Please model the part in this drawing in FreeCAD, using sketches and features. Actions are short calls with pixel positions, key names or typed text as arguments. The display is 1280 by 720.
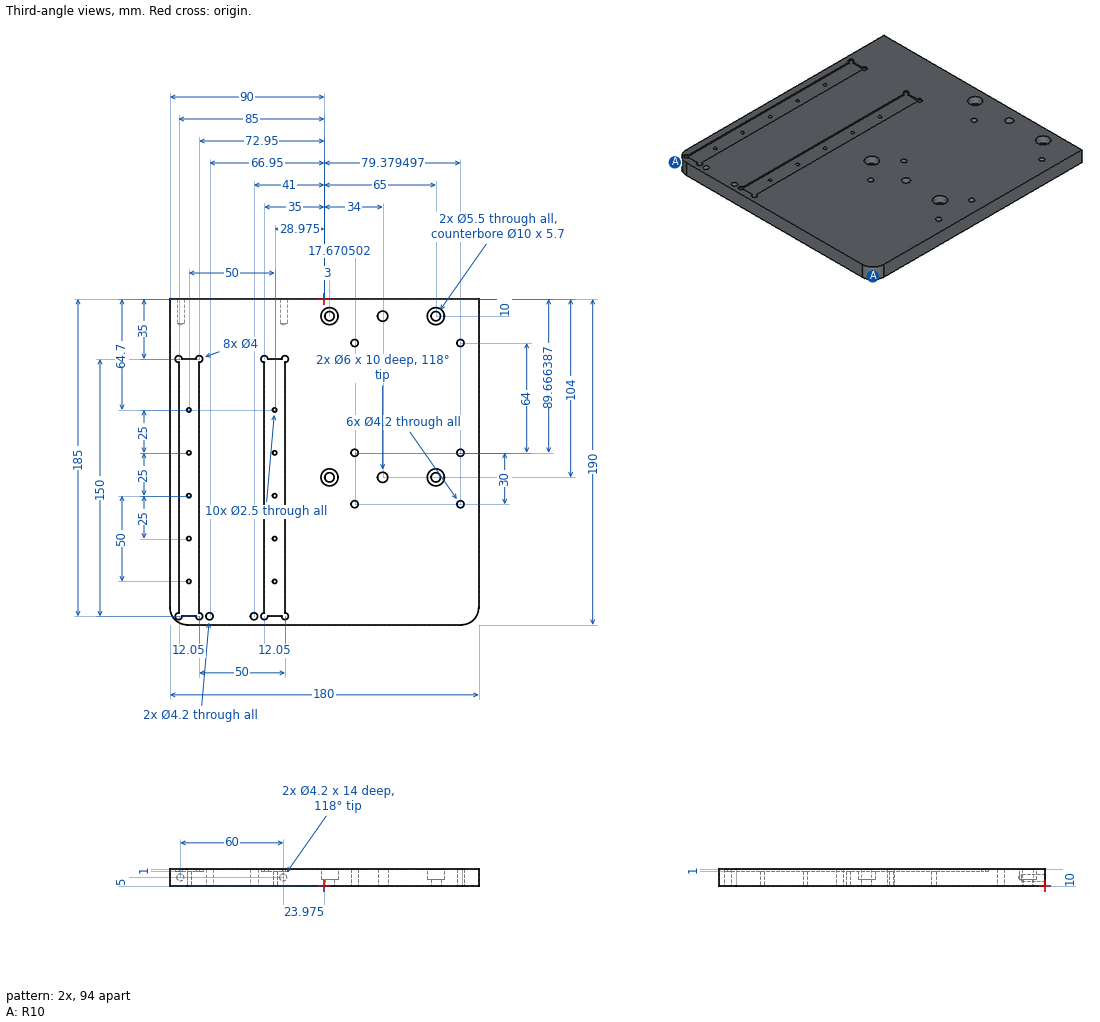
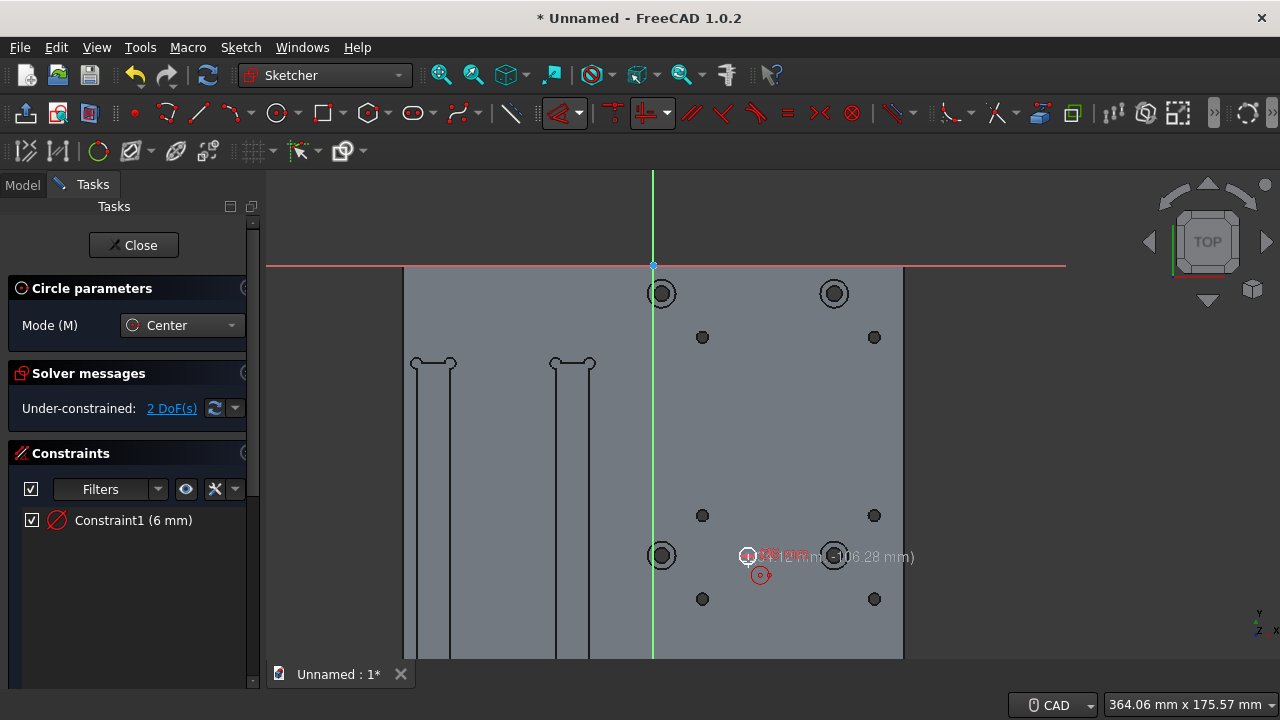
scroll(748, 294, up, 5)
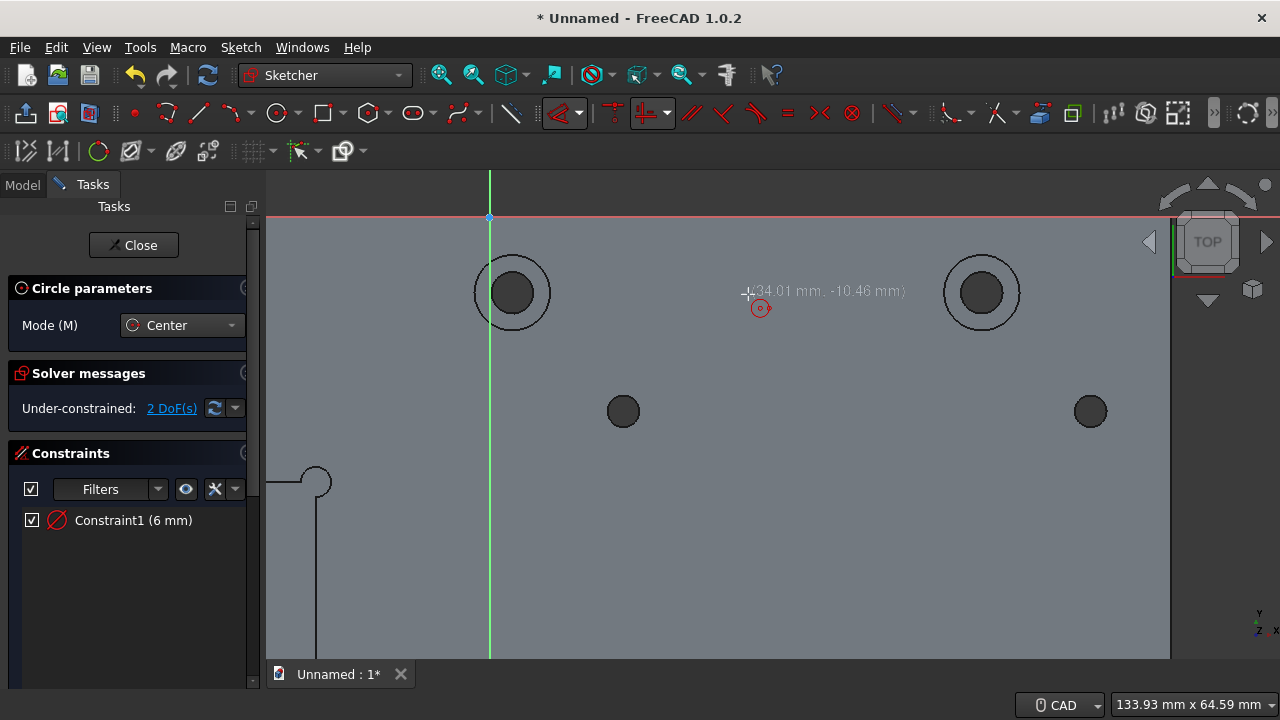
click(747, 293)
move(763, 277)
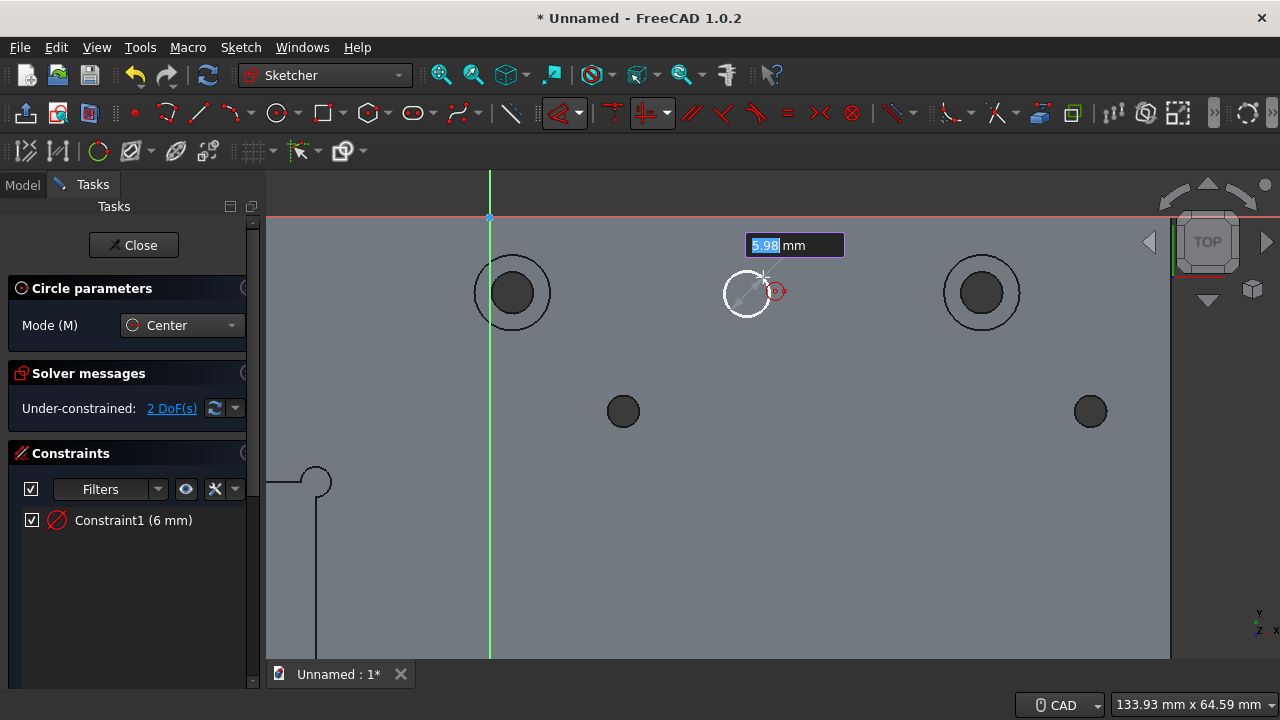
text(6)
key(Return)
key(Escape)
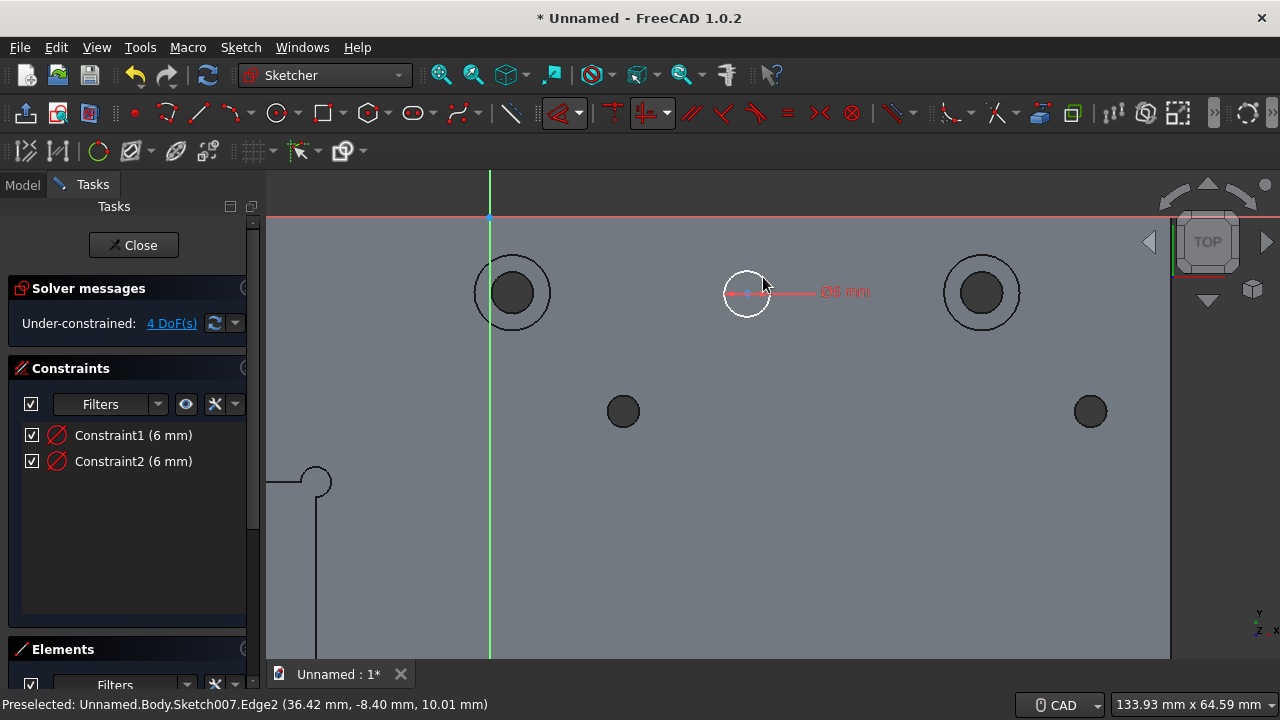
scroll(748, 294, down, 5)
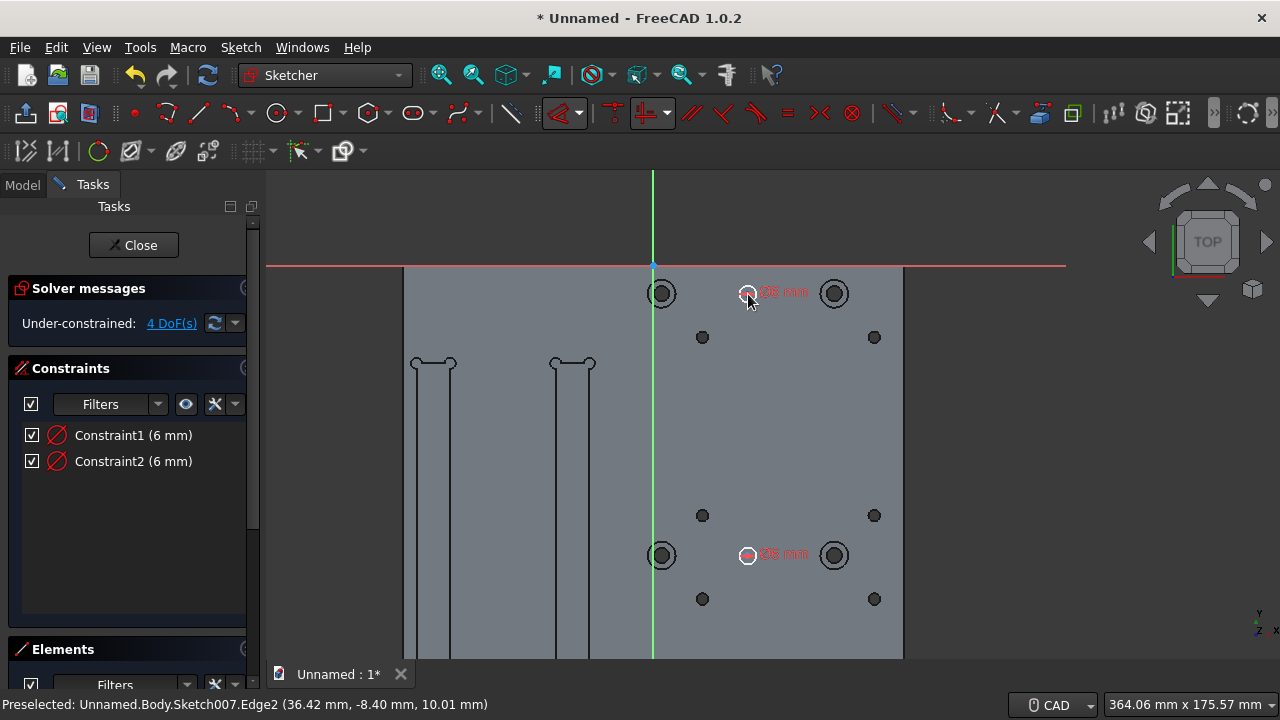
click(748, 556)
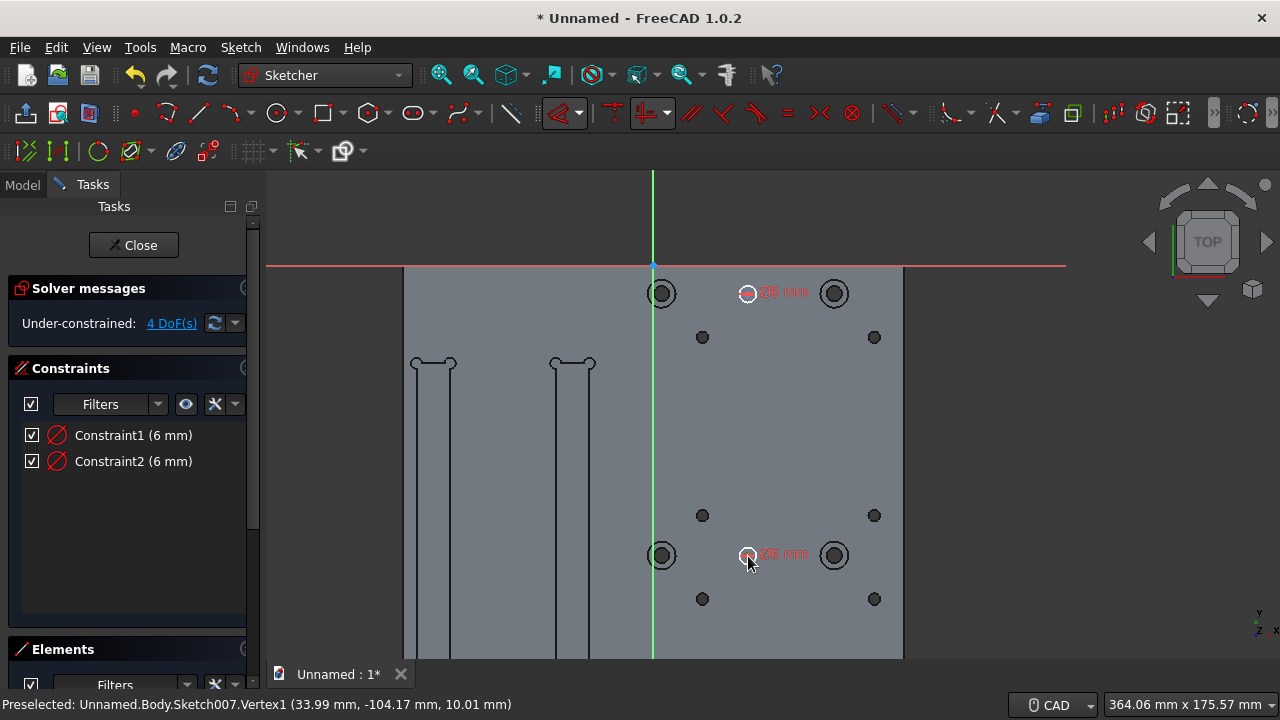
click(748, 294)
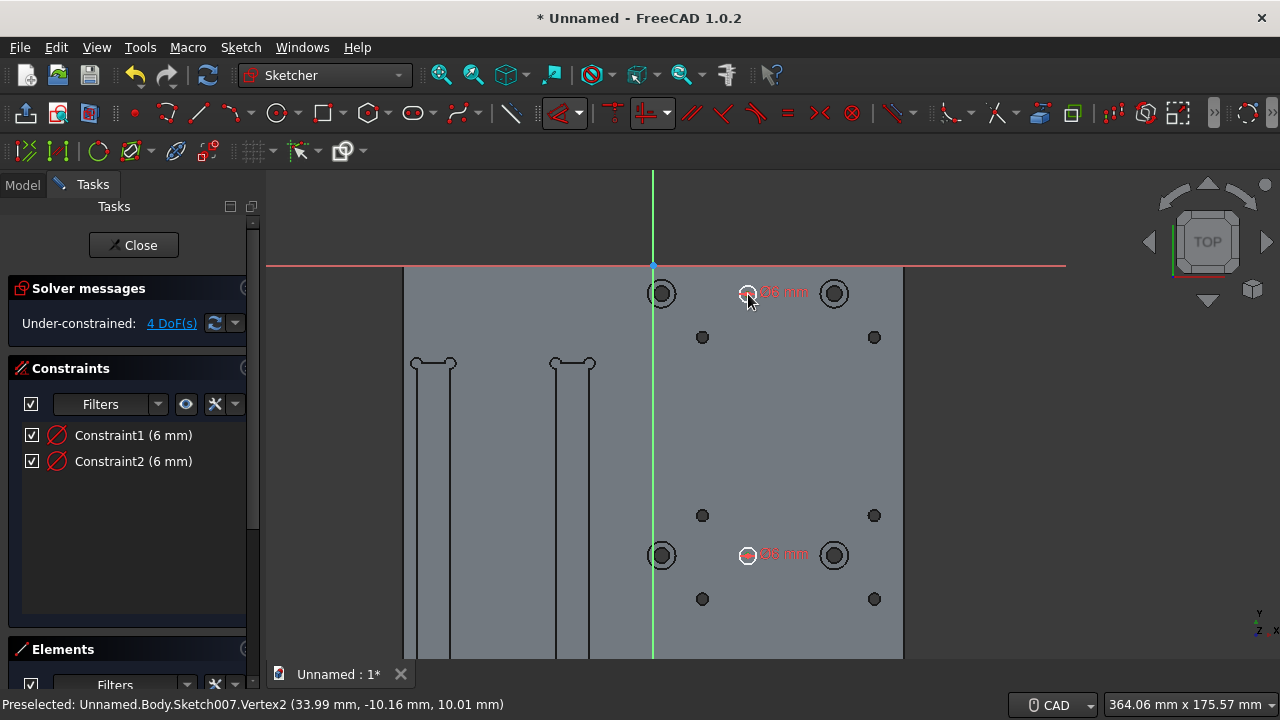
key(v)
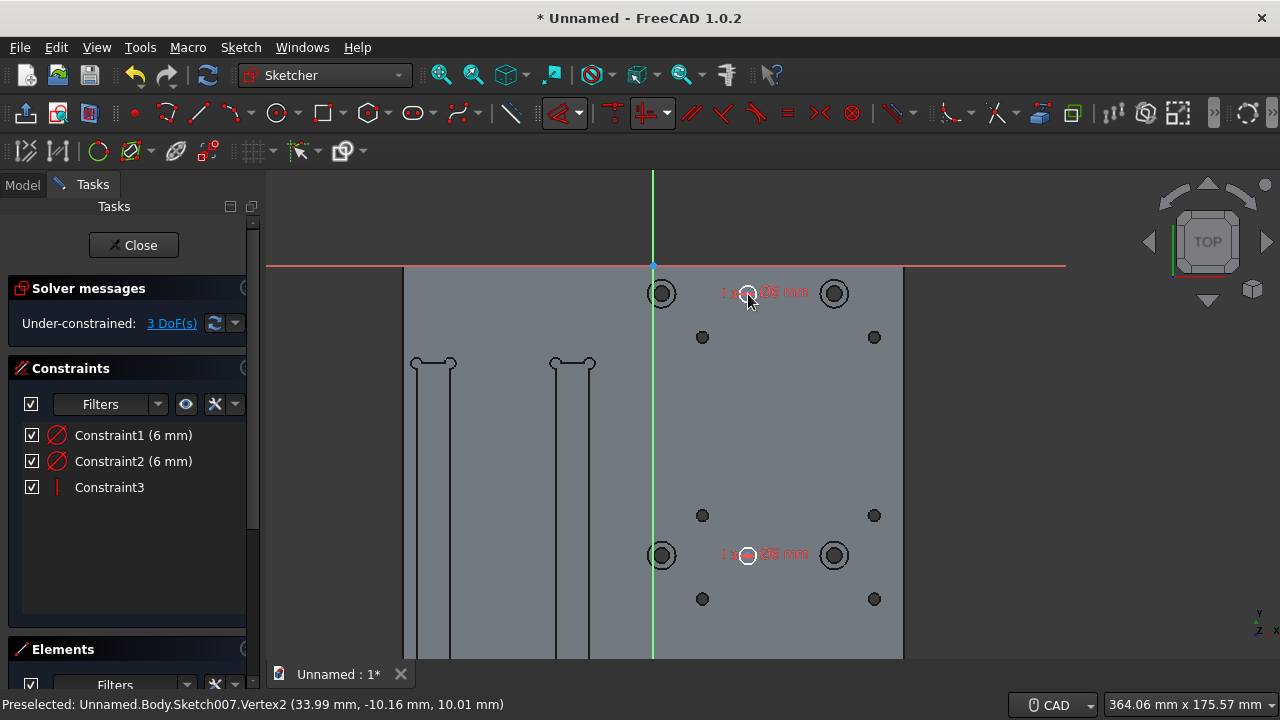
click(748, 556)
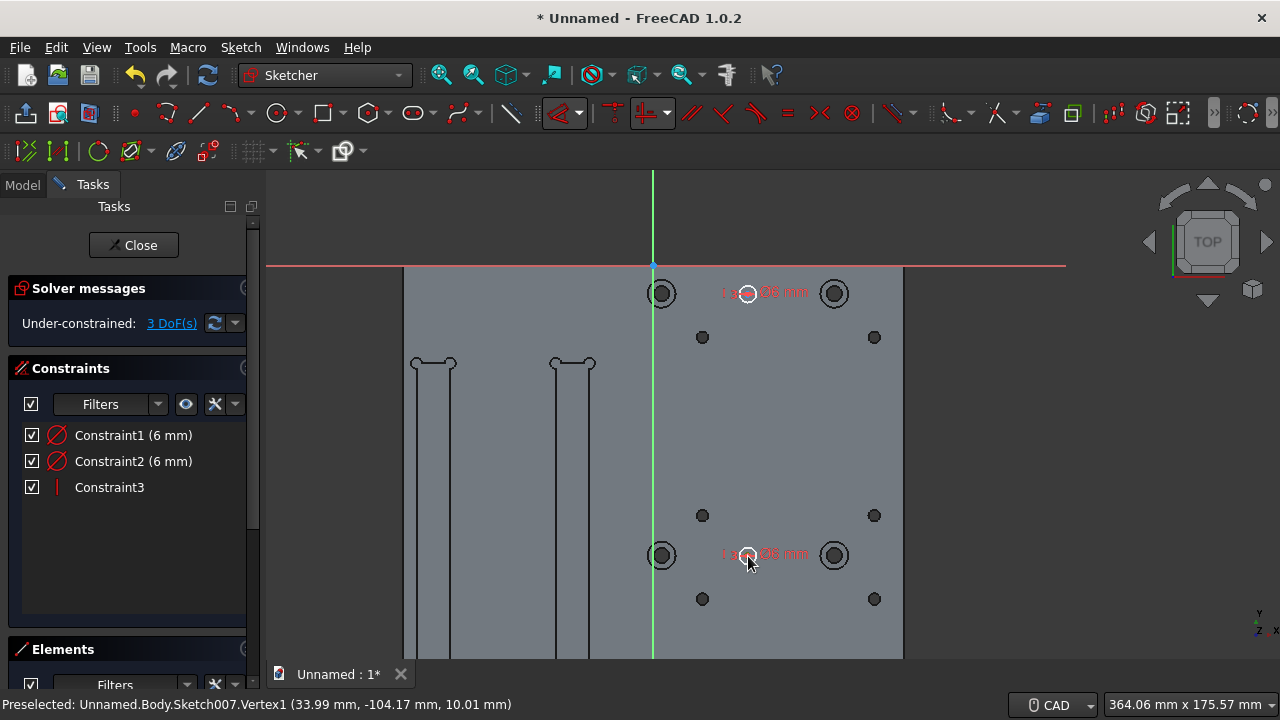
key(l)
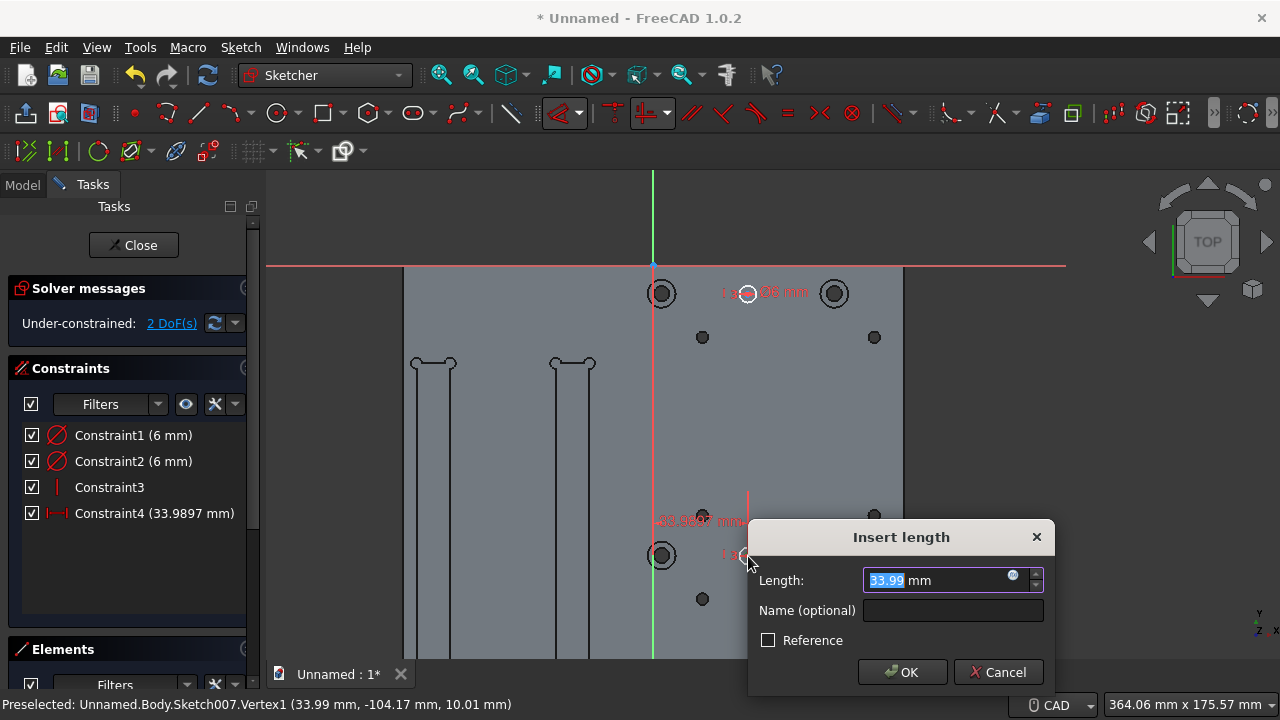
text(34)
key(Return)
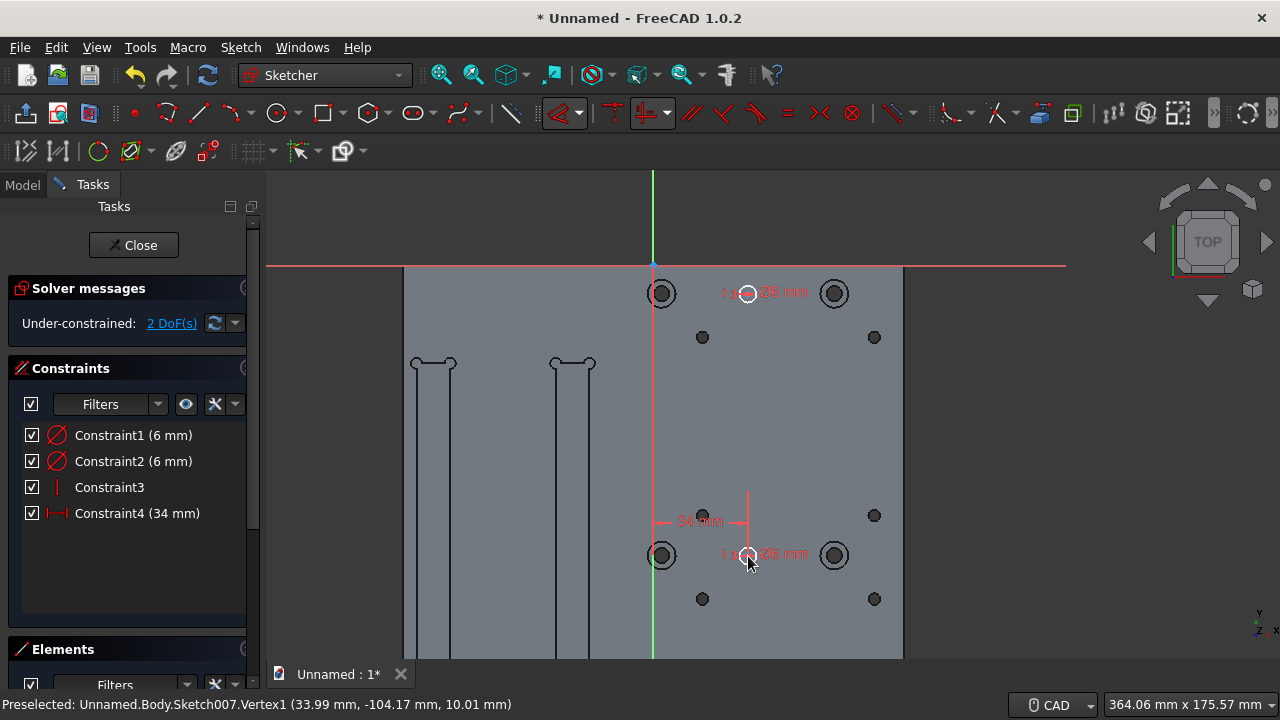
scroll(748, 294, up, 2)